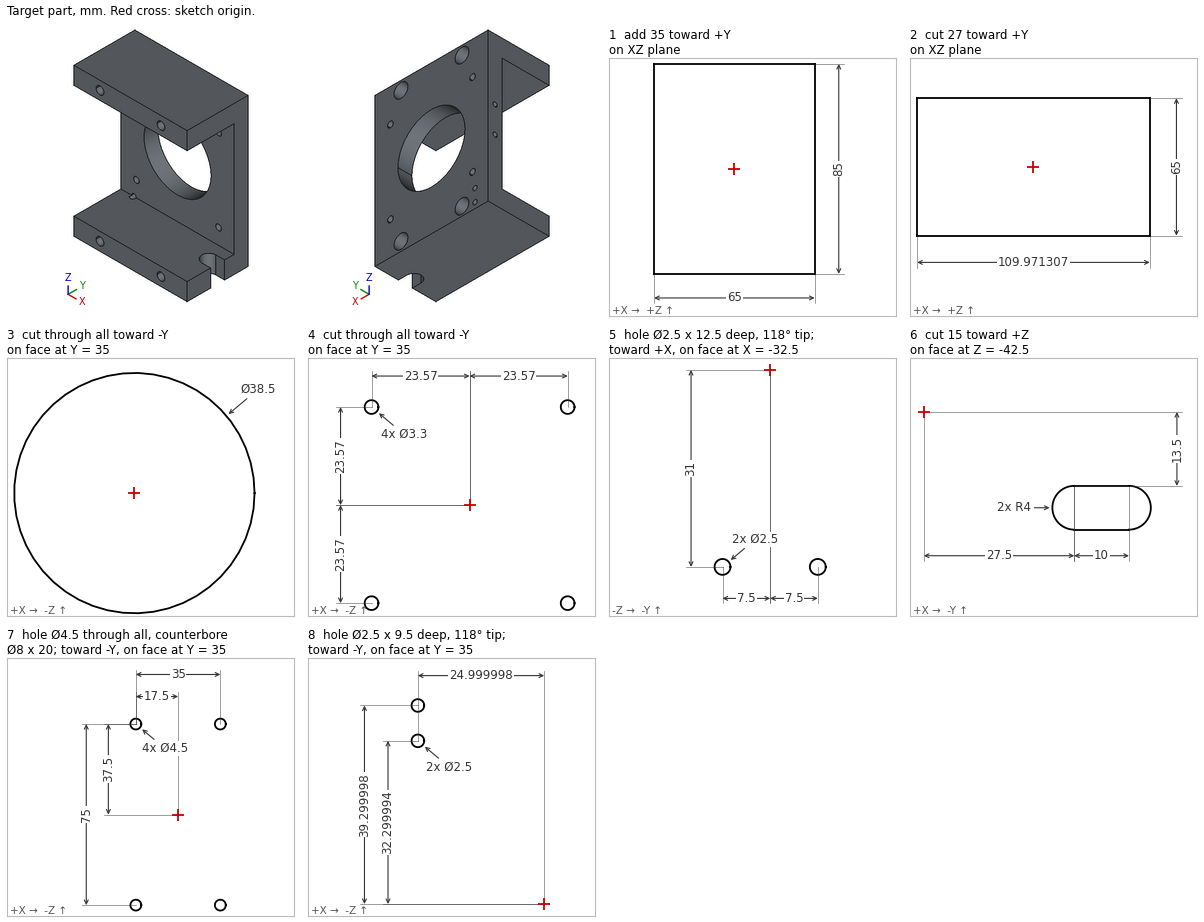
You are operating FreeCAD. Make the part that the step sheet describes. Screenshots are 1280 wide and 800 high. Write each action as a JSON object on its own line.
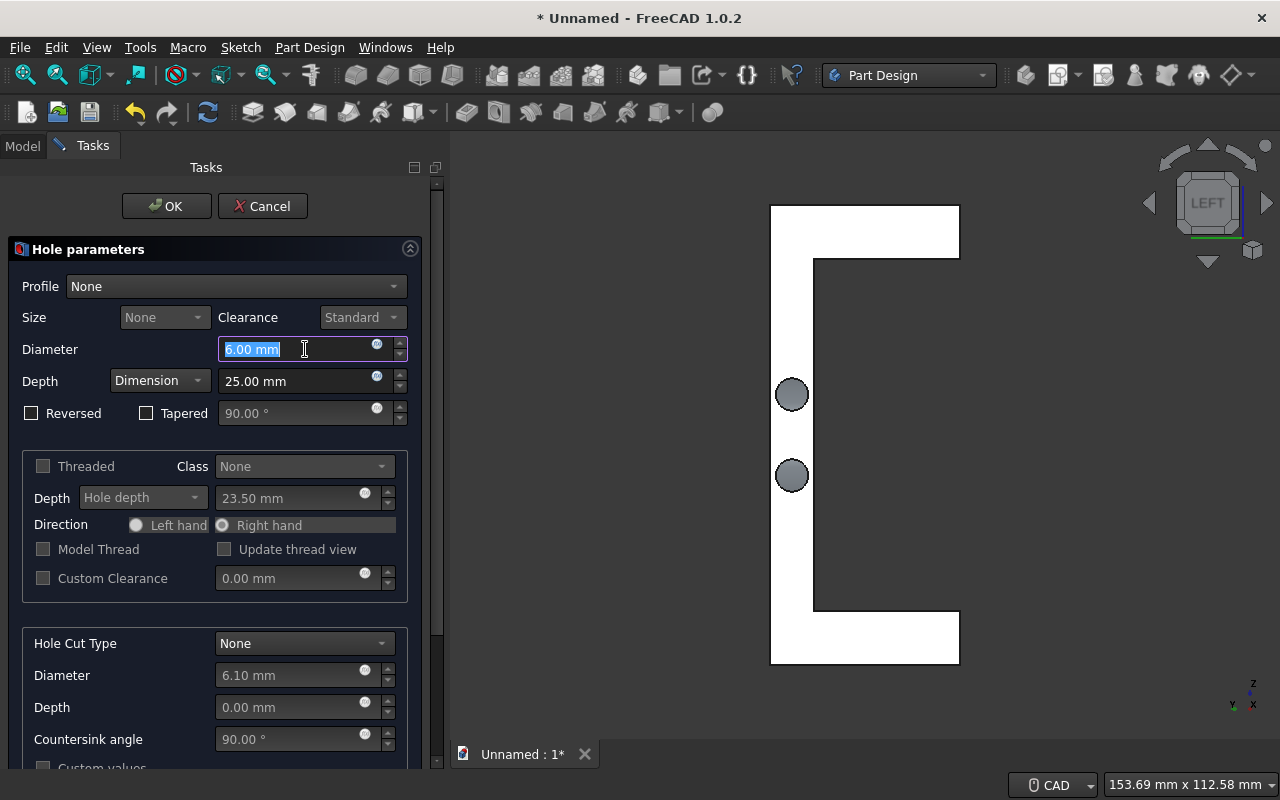
{"action": "type", "text": "2.5"}
{"action": "key", "text": "Tab"}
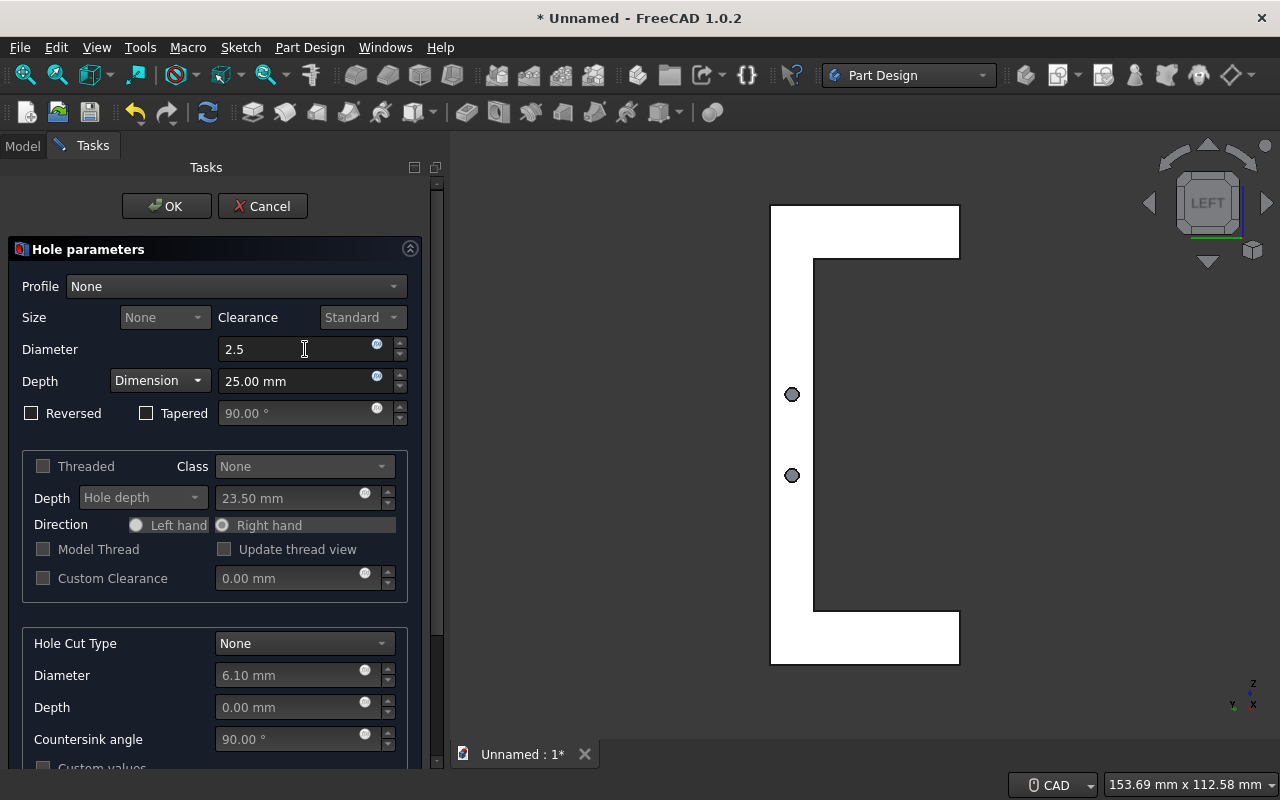
{"action": "triple_click", "coordinate": [305, 381]}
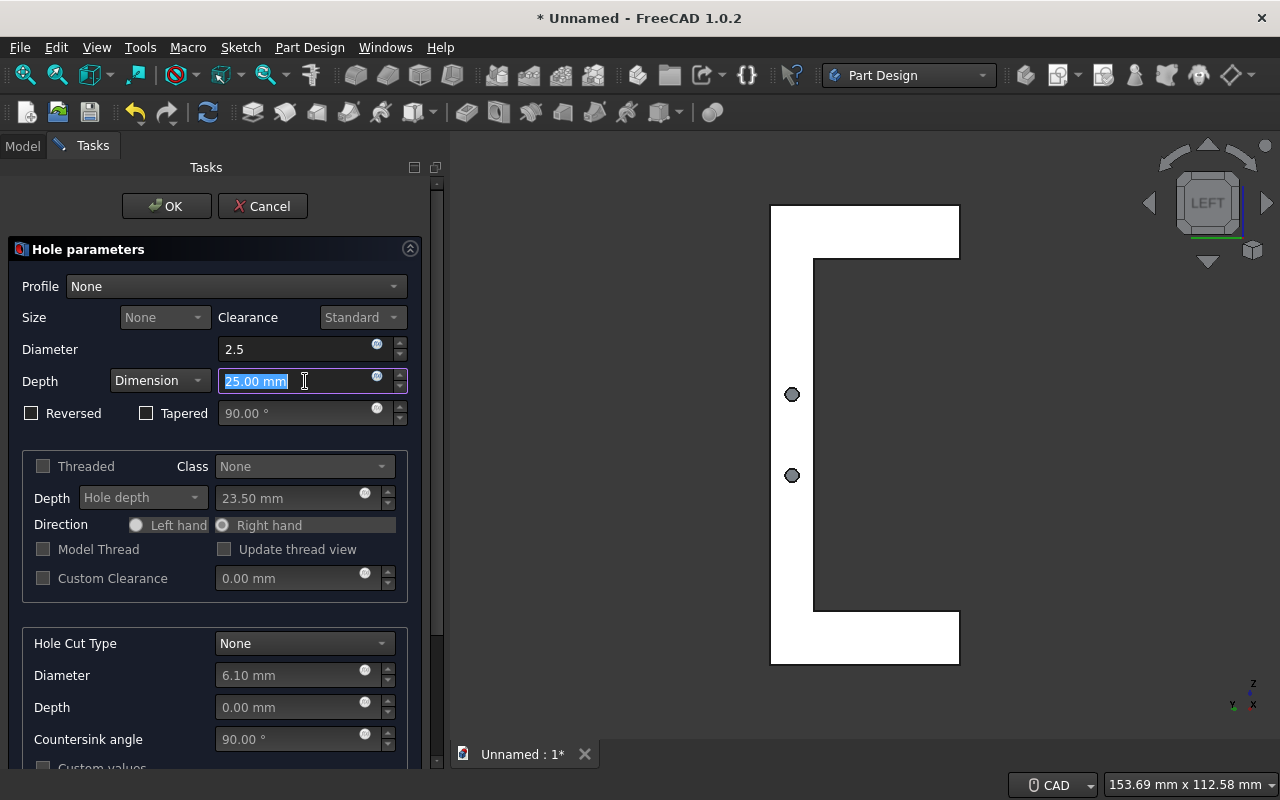
{"action": "type", "text": "12.5"}
{"action": "key", "text": "Tab"}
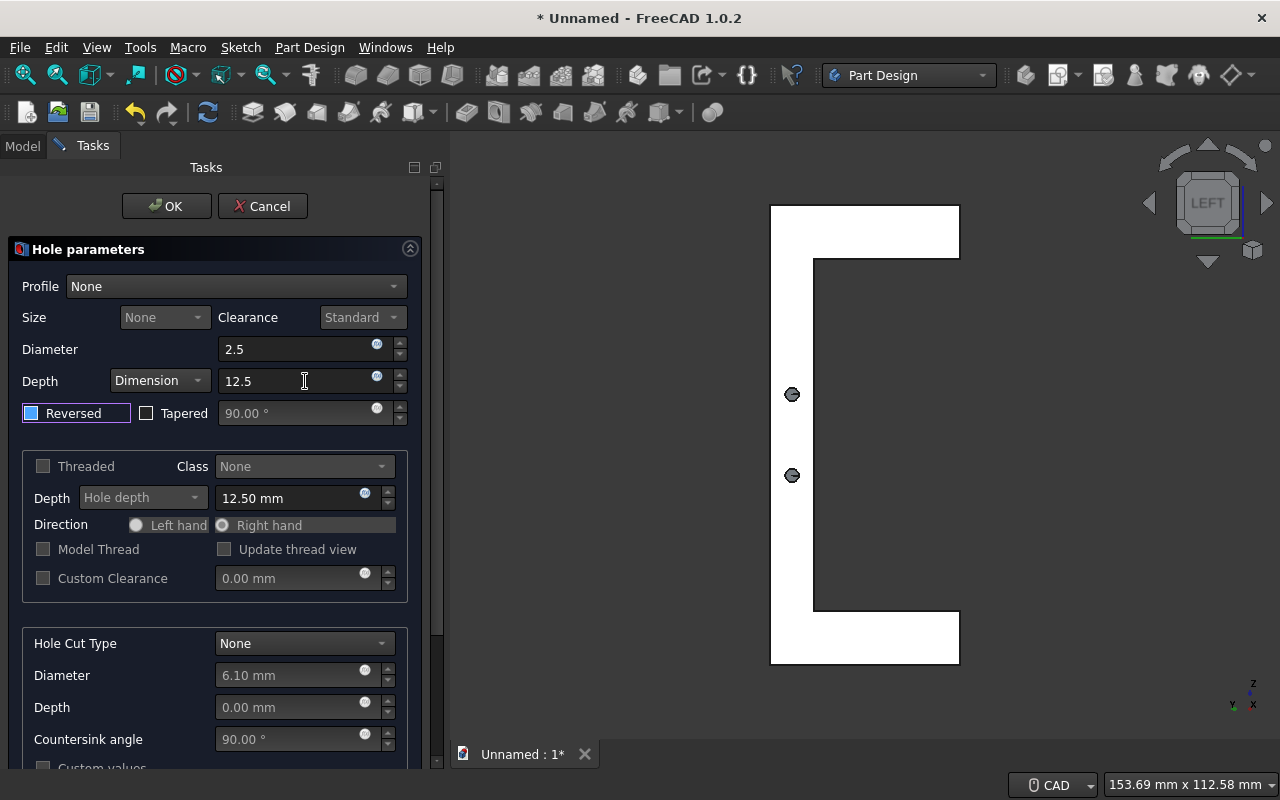
{"action": "left_click", "coordinate": [167, 206]}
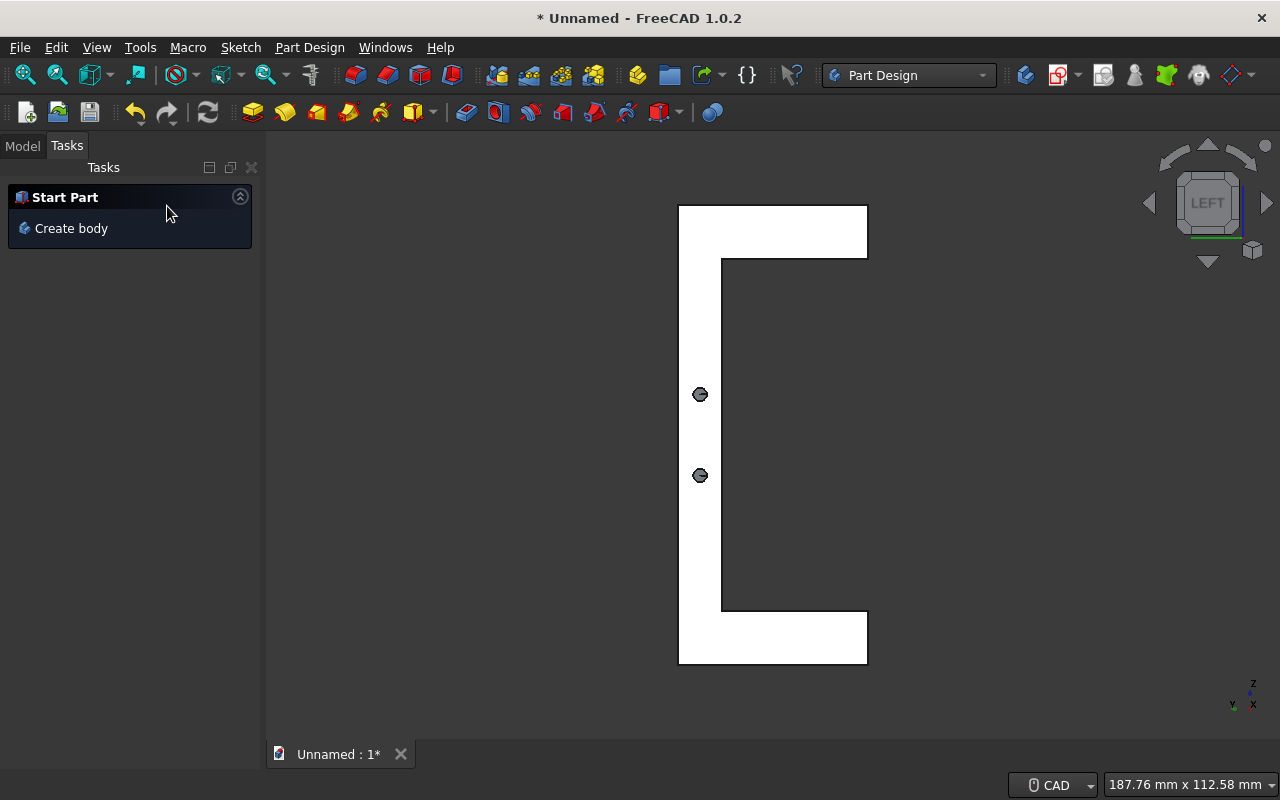
{"action": "key", "text": "5"}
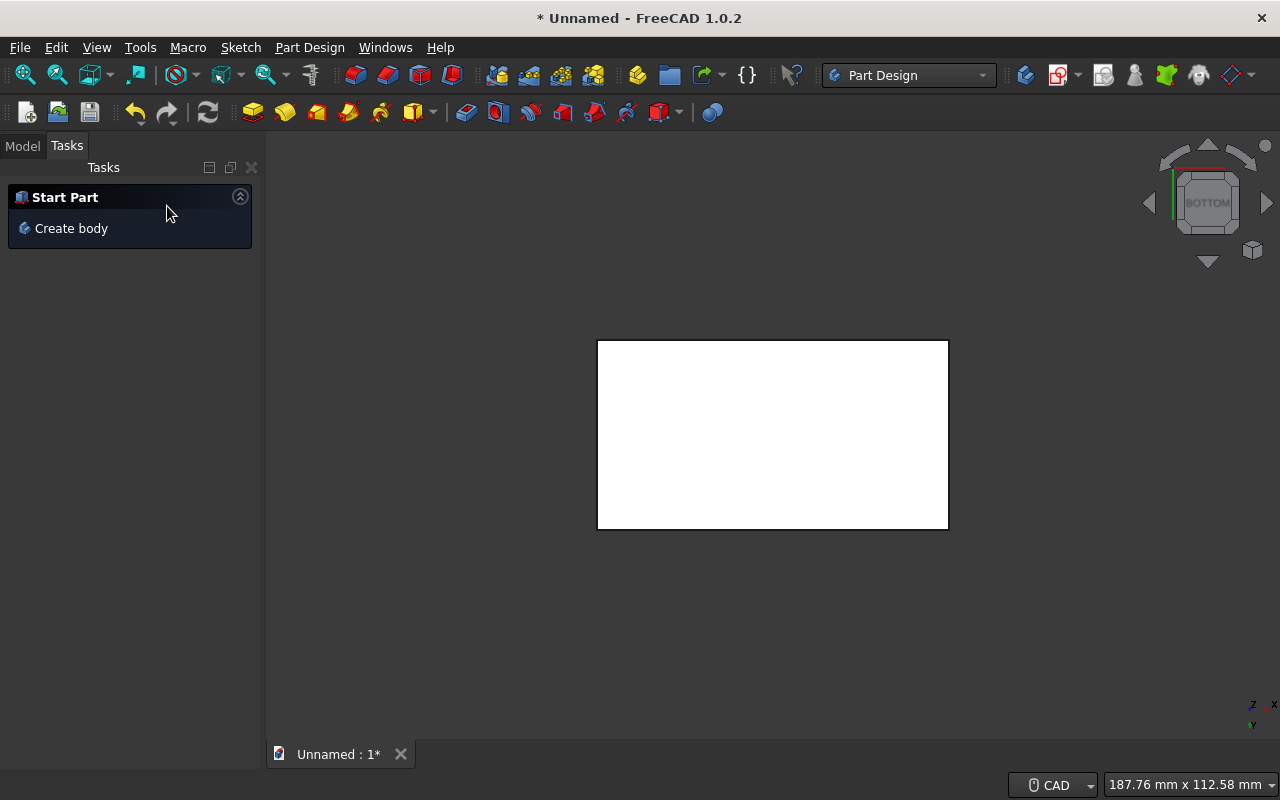
{"action": "left_click", "coordinate": [26, 76]}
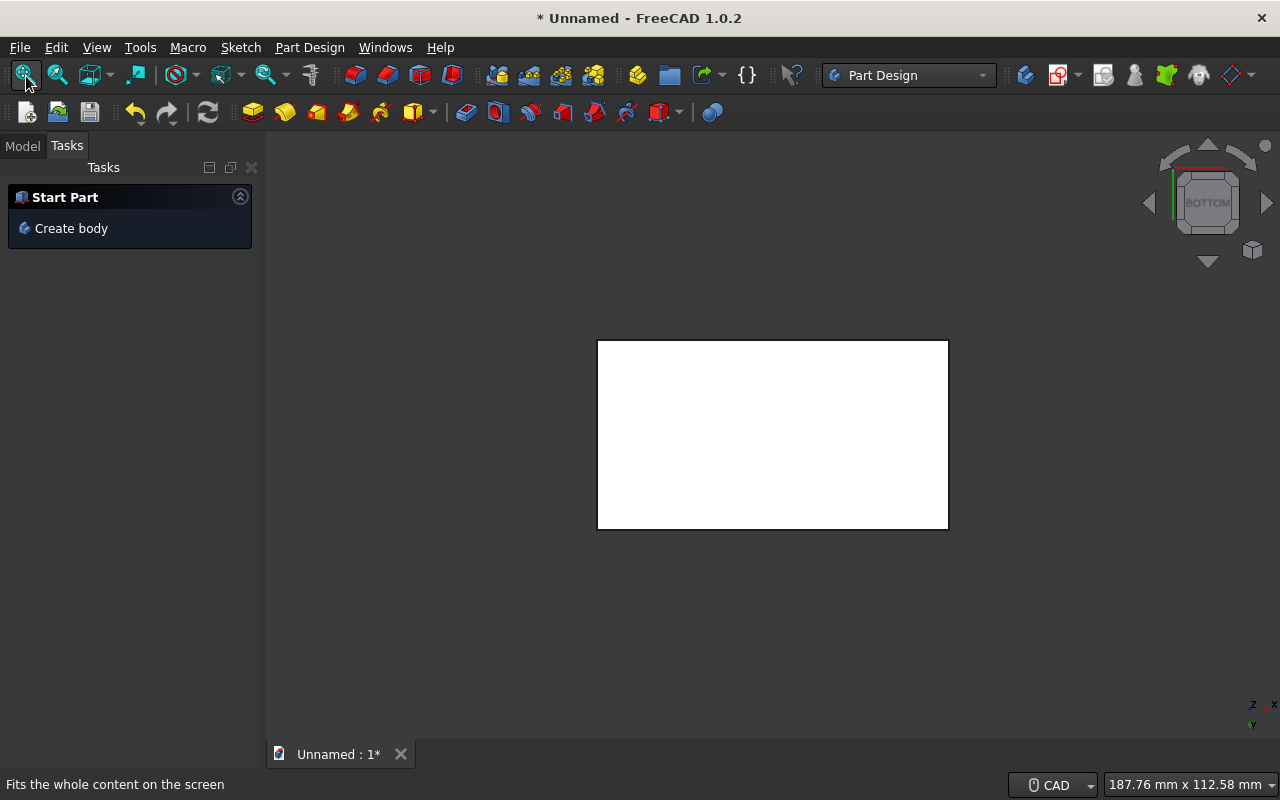
{"action": "left_click", "coordinate": [823, 434]}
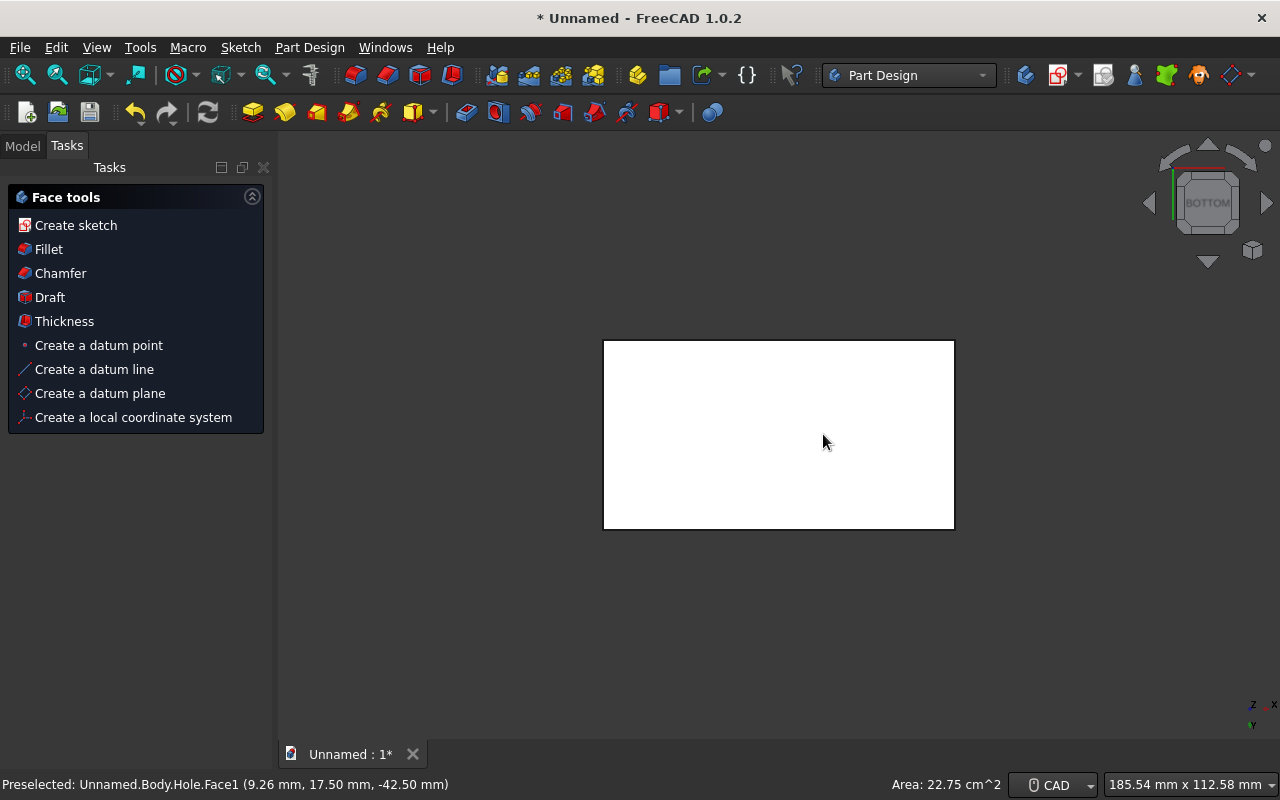
{"action": "left_click", "coordinate": [1058, 76]}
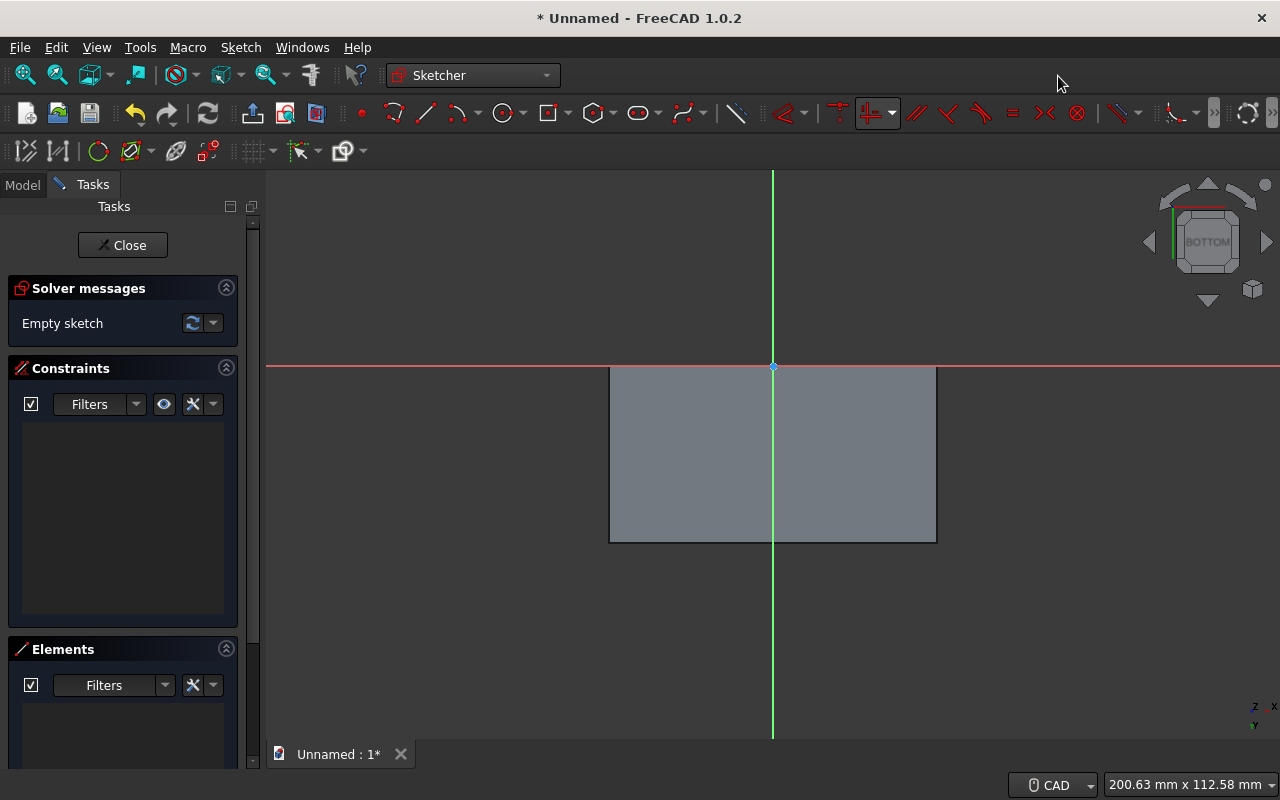
{"action": "scroll", "coordinate": [979, 401], "scroll_direction": "up", "scroll_amount": 5}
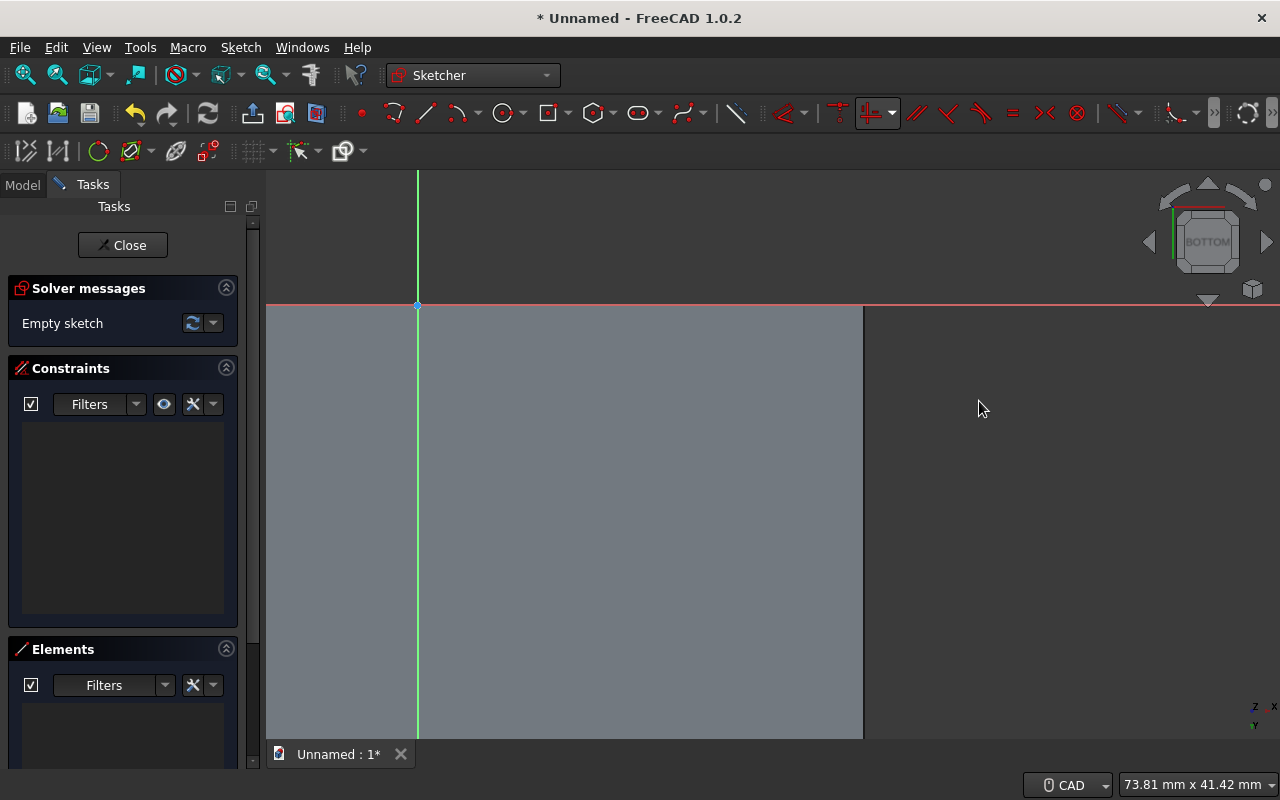
{"action": "left_click", "coordinate": [638, 114]}